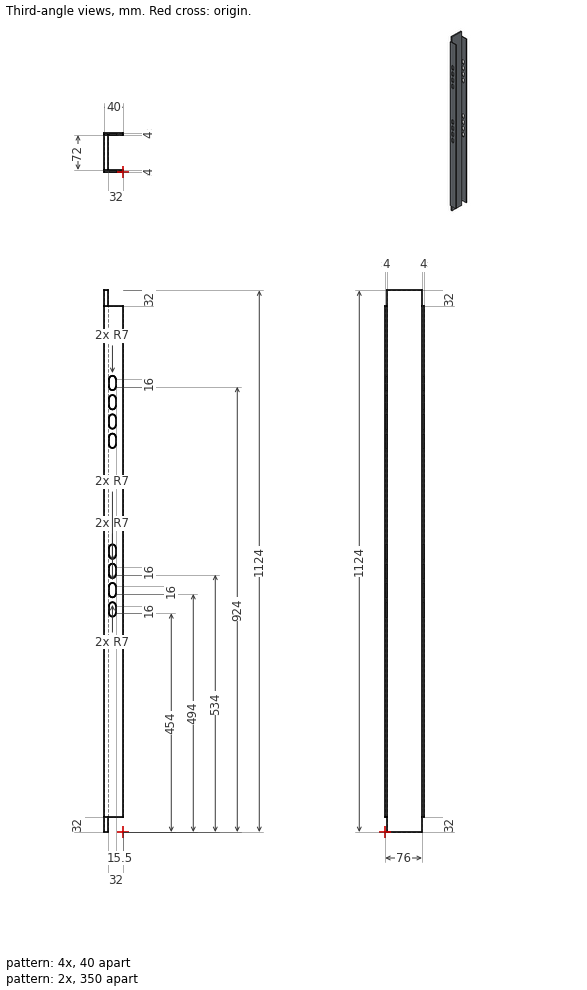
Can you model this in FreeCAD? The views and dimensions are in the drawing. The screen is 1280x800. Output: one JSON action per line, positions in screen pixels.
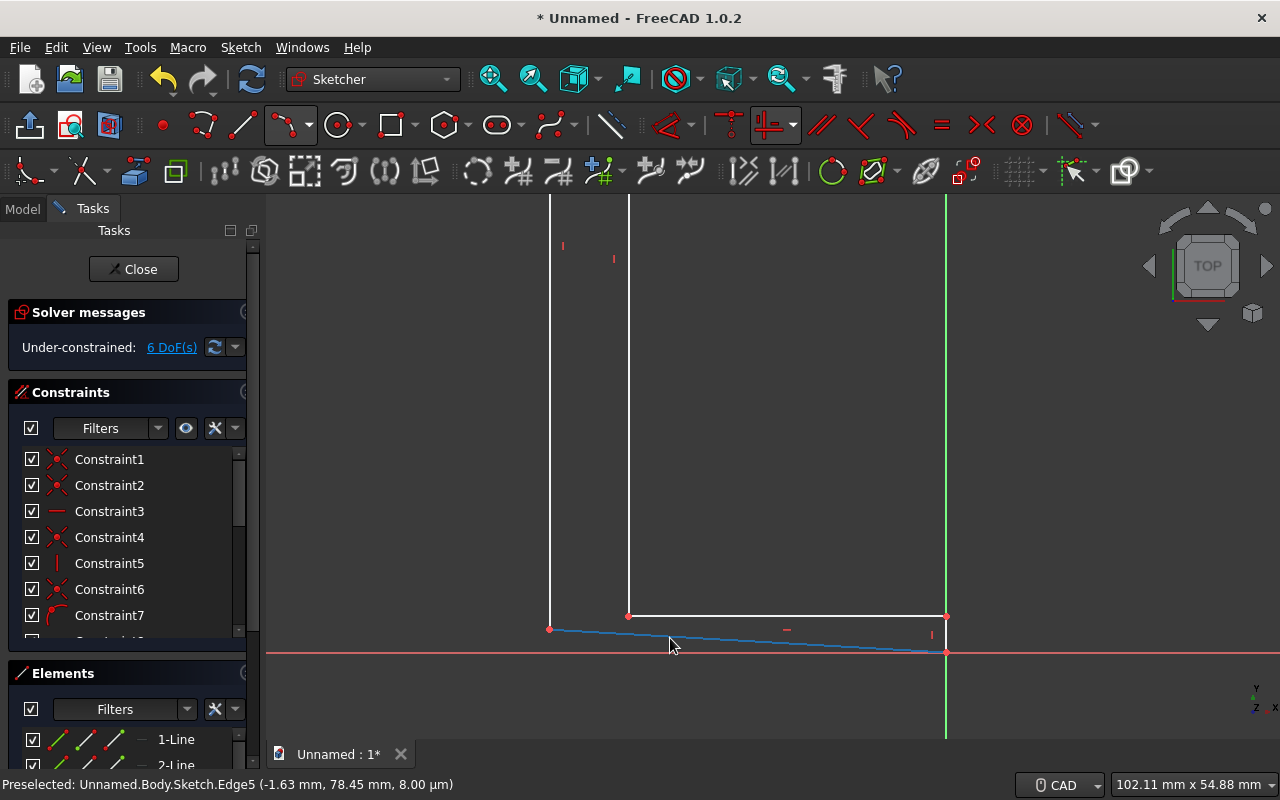
{"action": "left_click", "coordinate": [669, 637]}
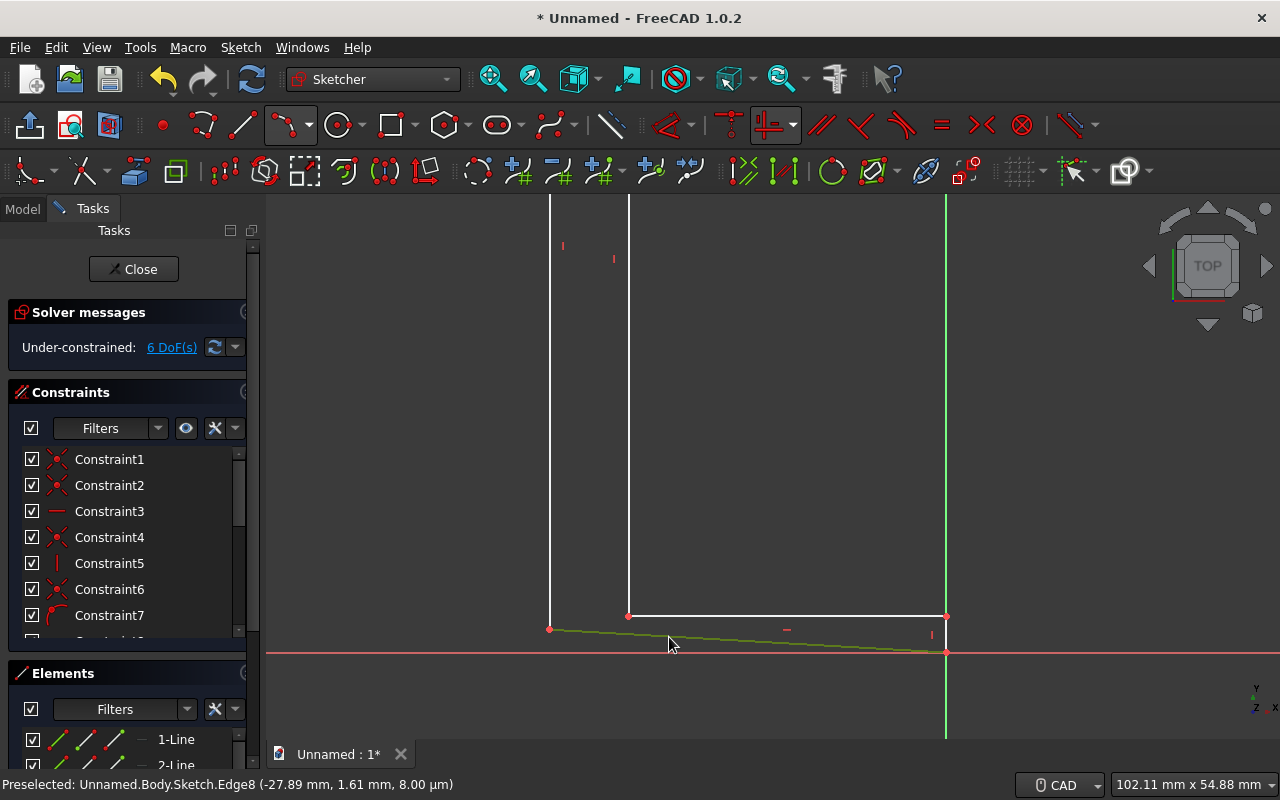
{"action": "key", "text": "h"}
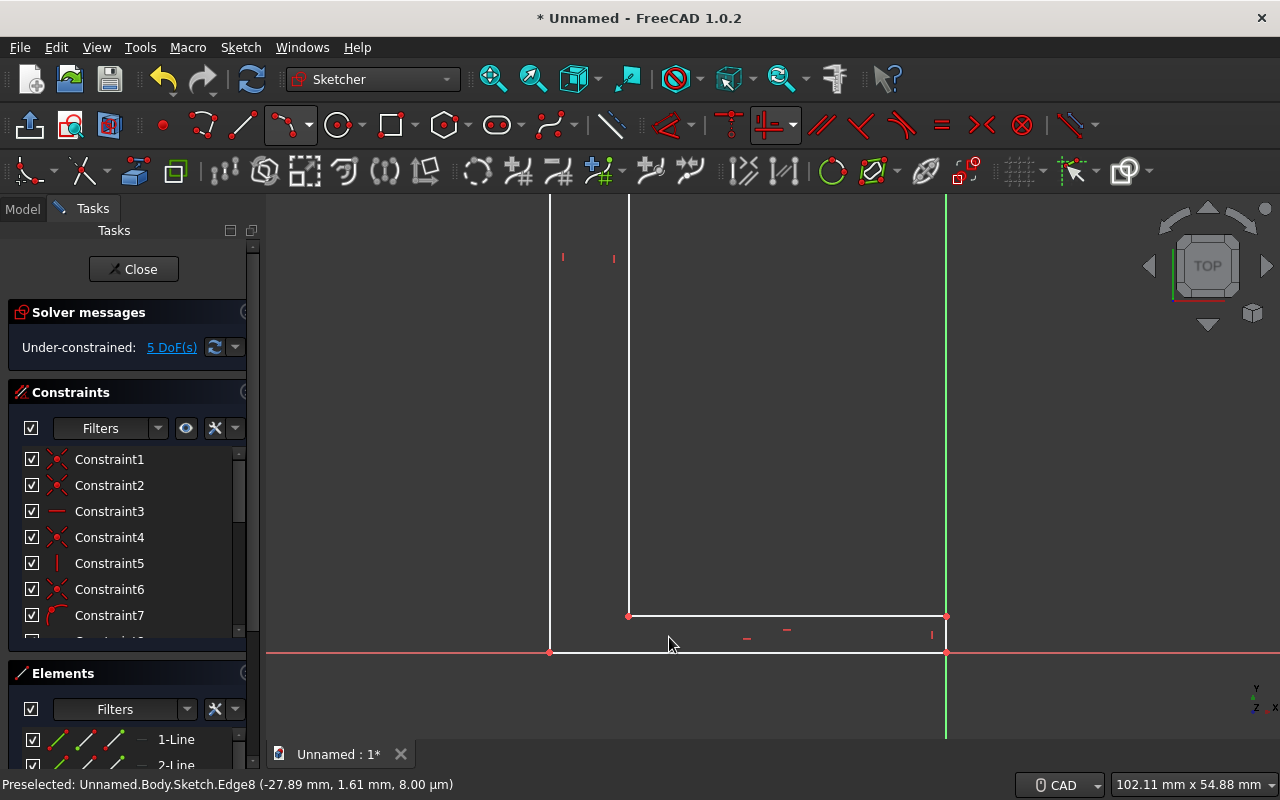
{"action": "left_click", "coordinate": [666, 126]}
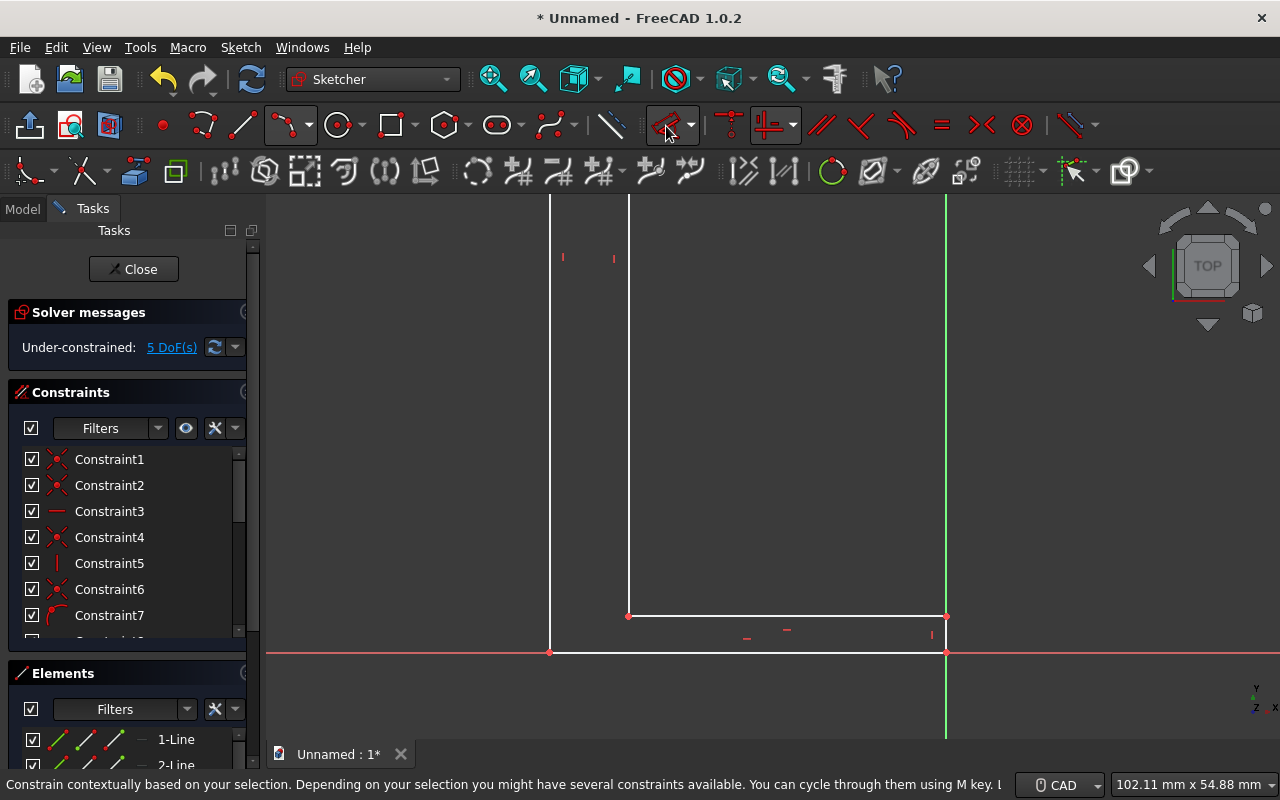
{"action": "scroll", "coordinate": [946, 642], "scroll_direction": "up", "scroll_amount": 2}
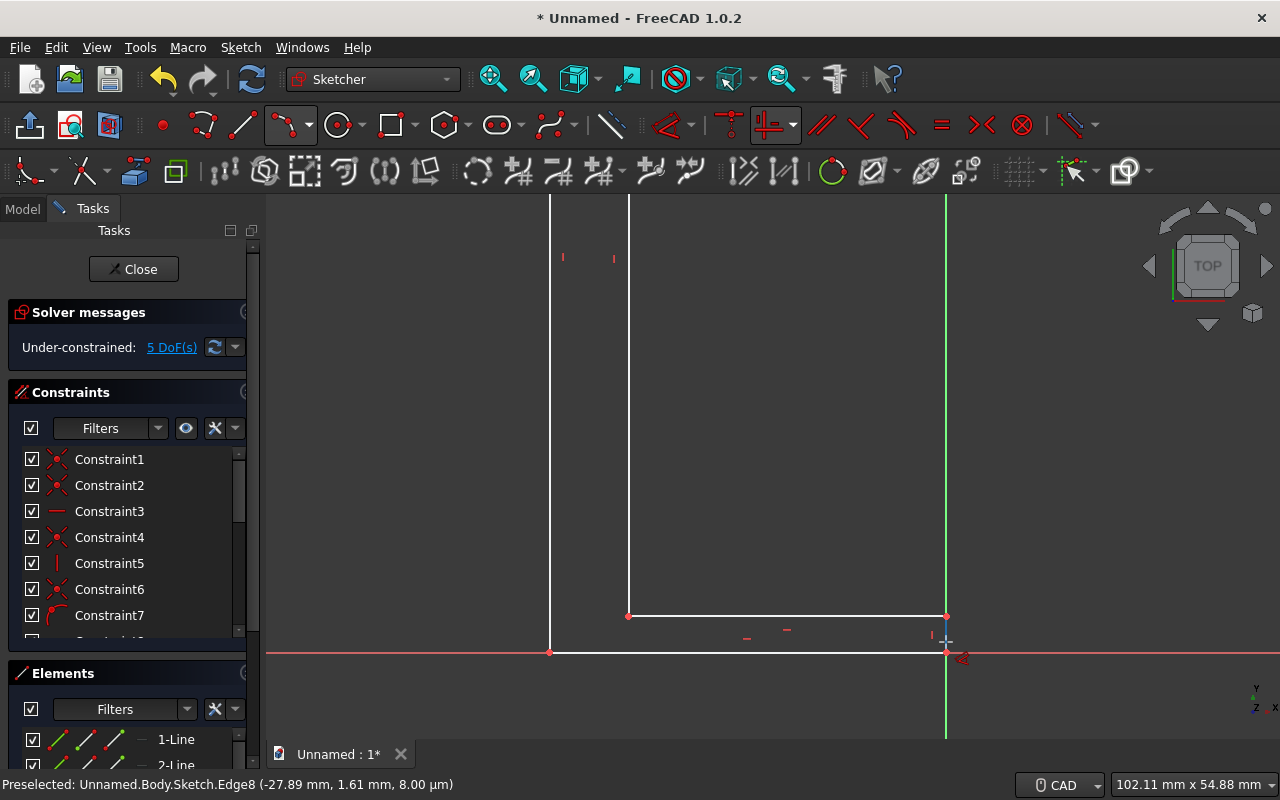
{"action": "left_click", "coordinate": [946, 641]}
{"action": "left_click", "coordinate": [980, 630]}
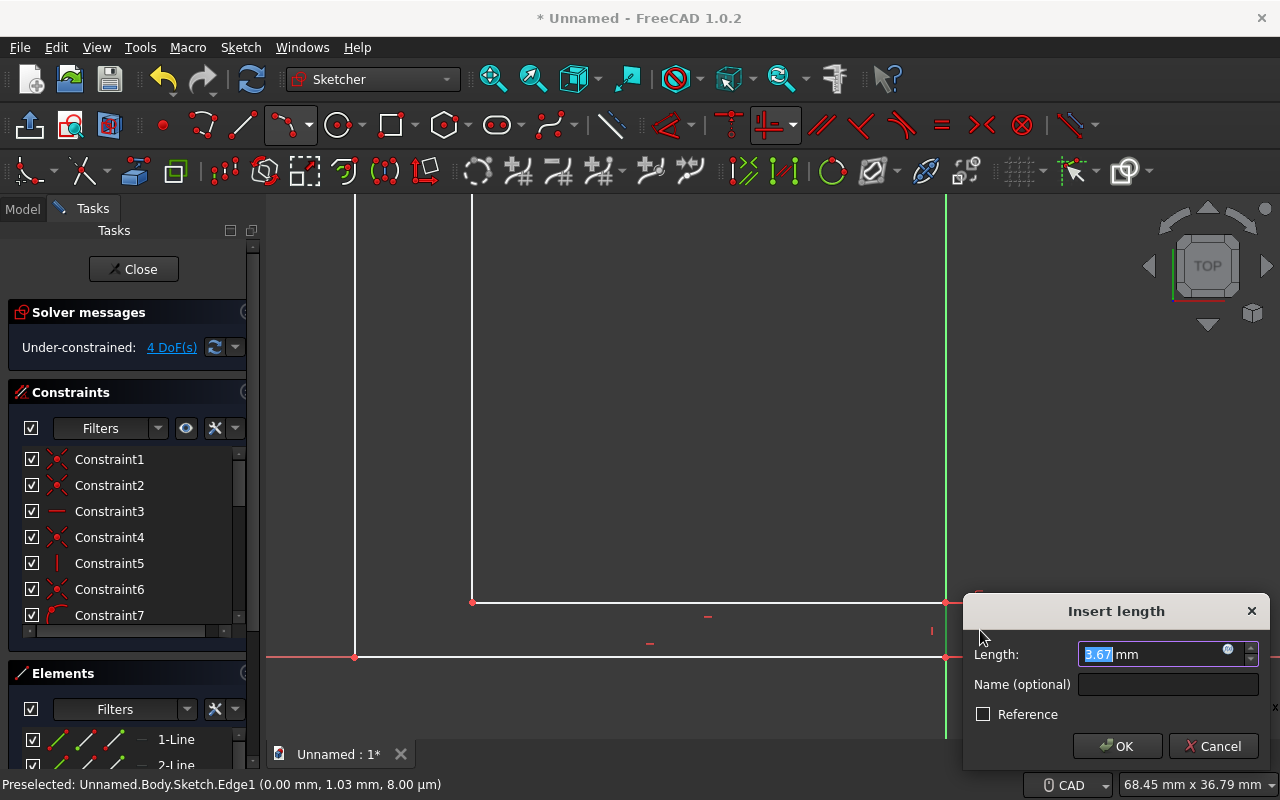
{"action": "type", "text": "4"}
{"action": "key", "text": "Return"}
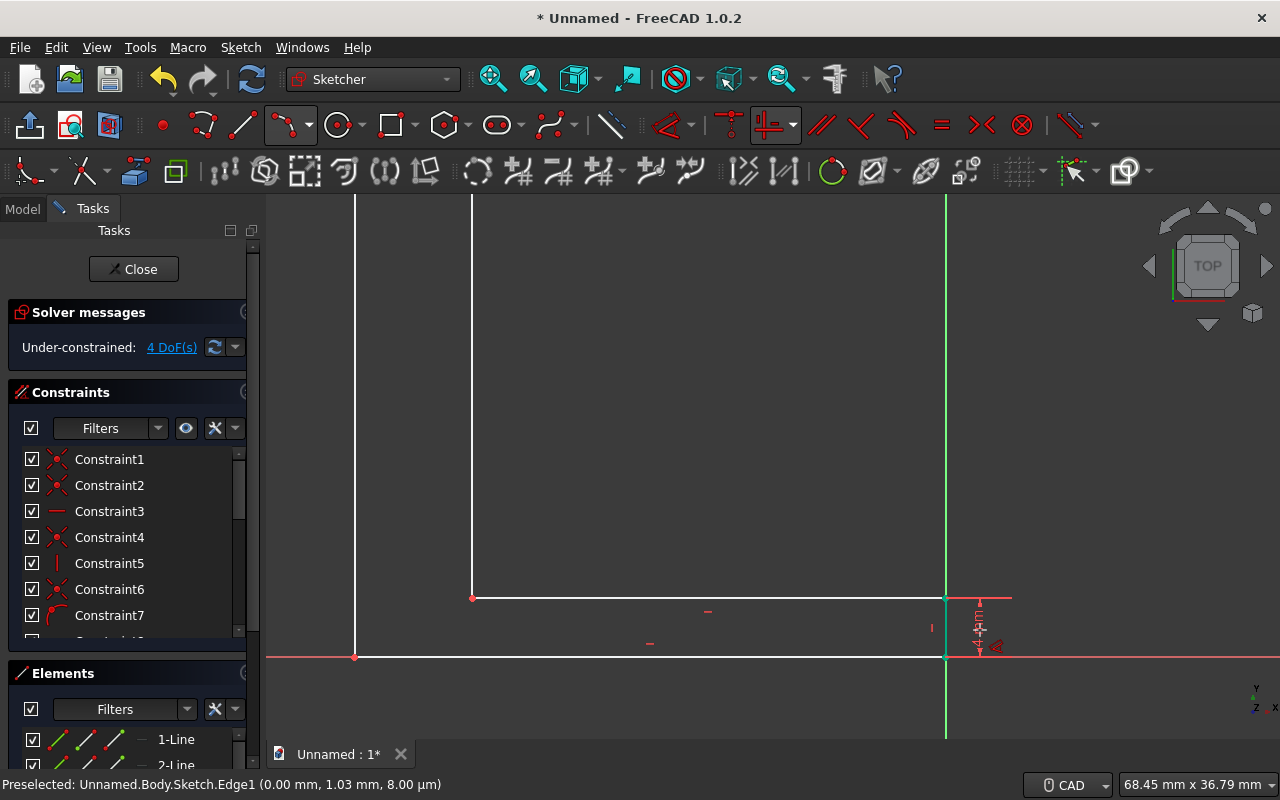
{"action": "scroll", "coordinate": [728, 640], "scroll_direction": "down", "scroll_amount": 6}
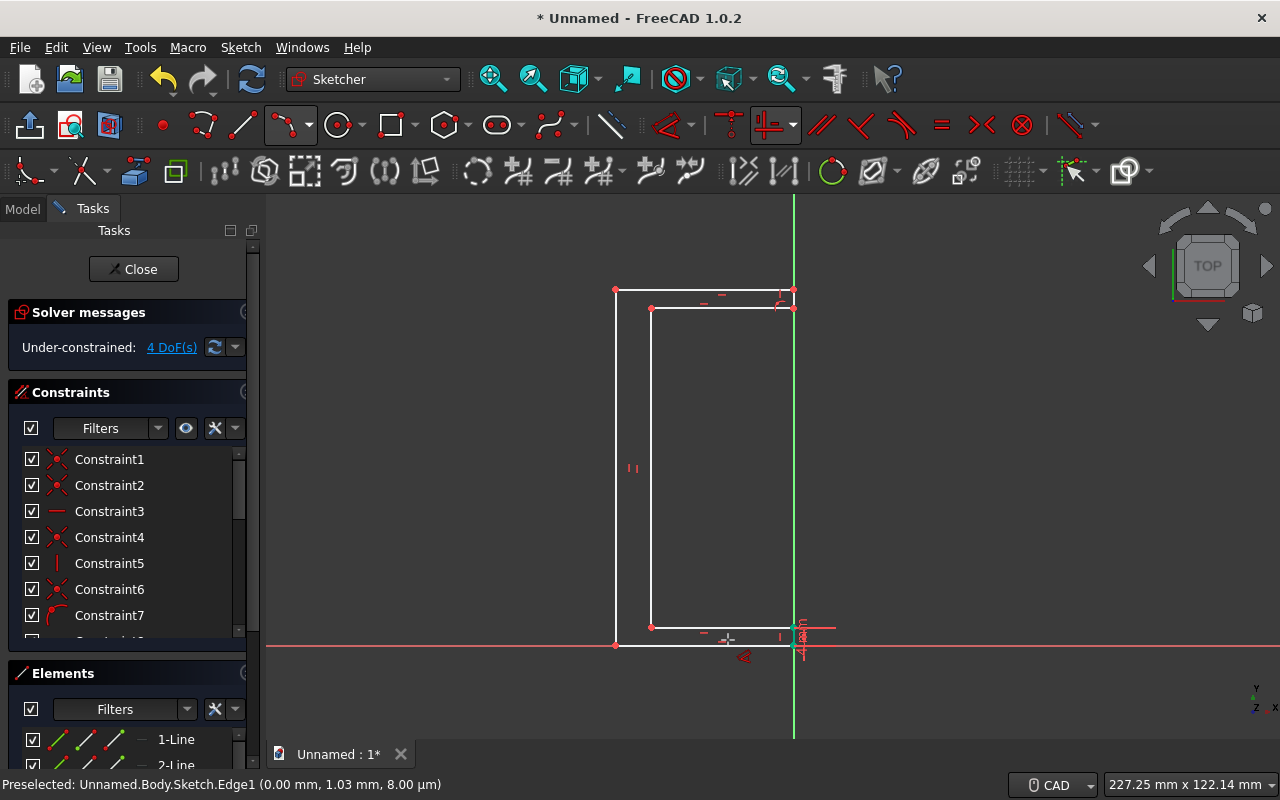
{"action": "scroll", "coordinate": [794, 303], "scroll_direction": "up", "scroll_amount": 5}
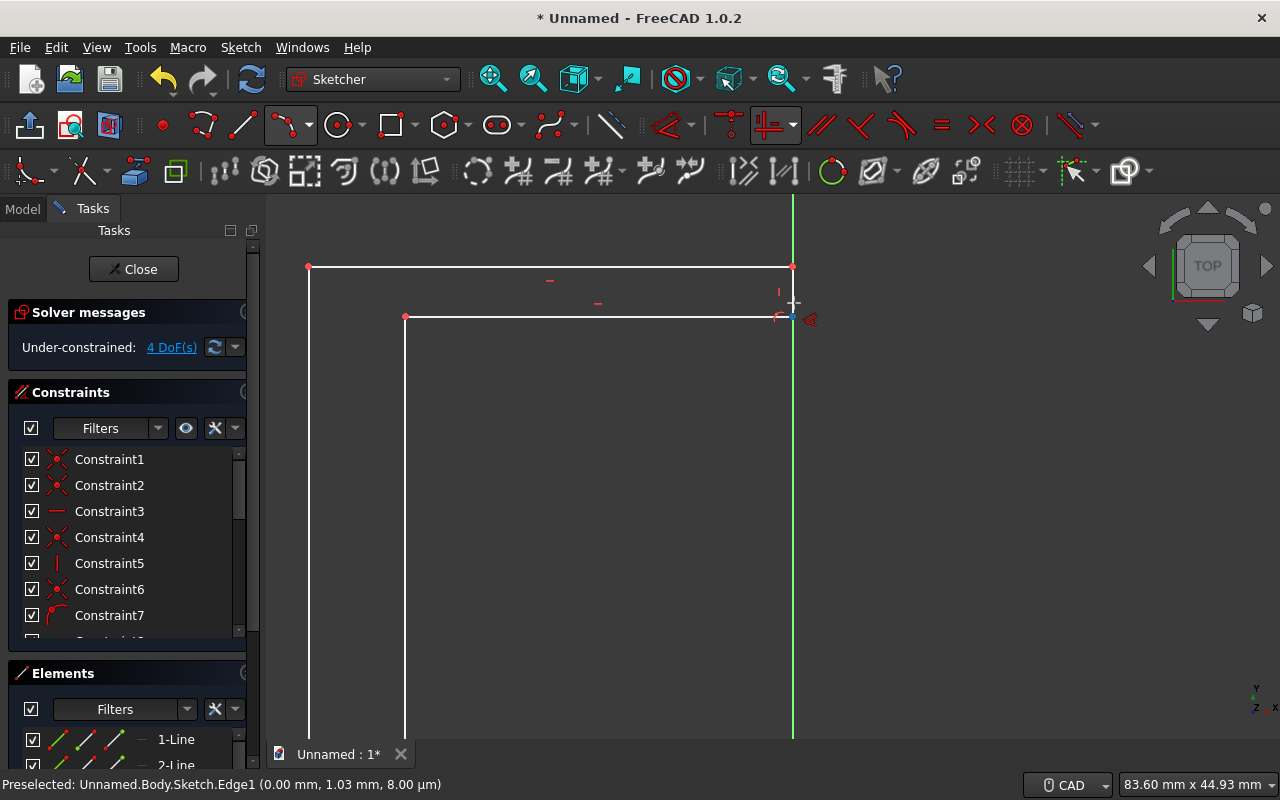
{"action": "left_click", "coordinate": [793, 302]}
{"action": "left_click", "coordinate": [827, 292]}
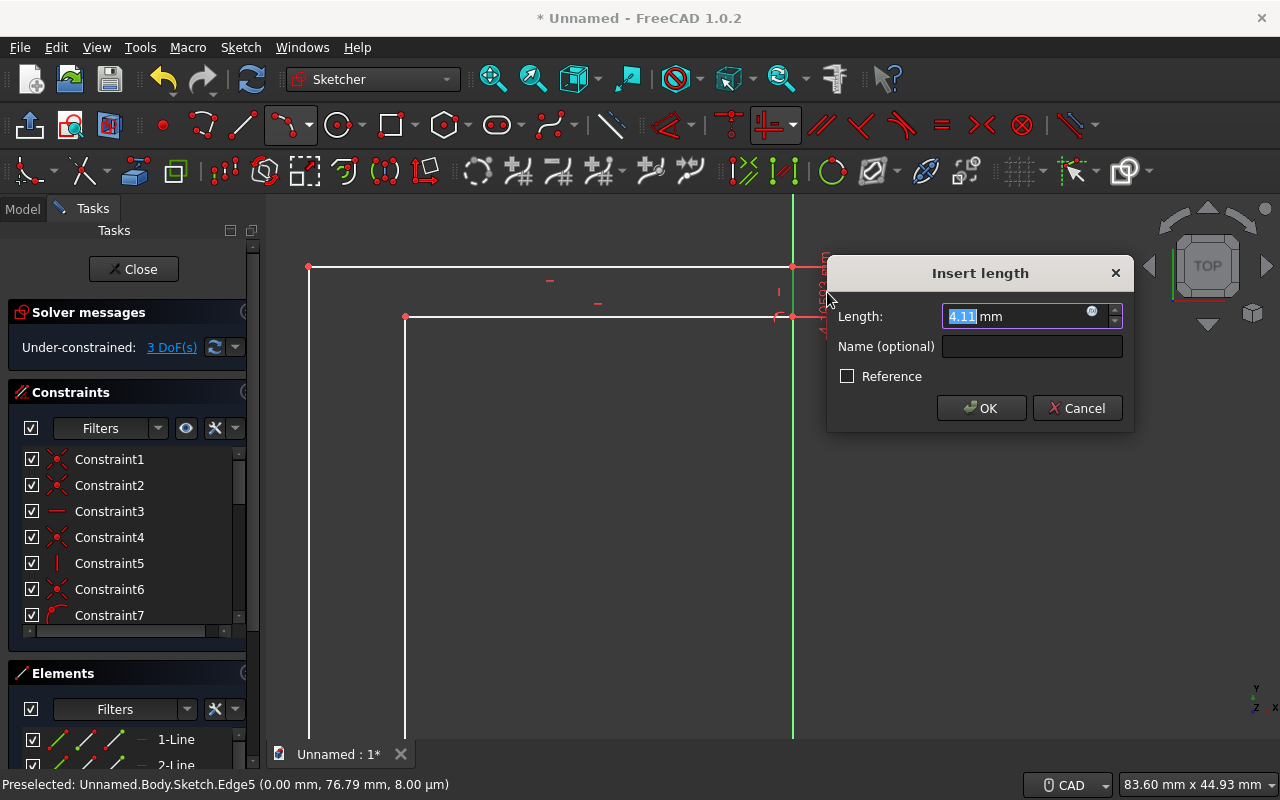
{"action": "type", "text": "4"}
{"action": "key", "text": "Return"}